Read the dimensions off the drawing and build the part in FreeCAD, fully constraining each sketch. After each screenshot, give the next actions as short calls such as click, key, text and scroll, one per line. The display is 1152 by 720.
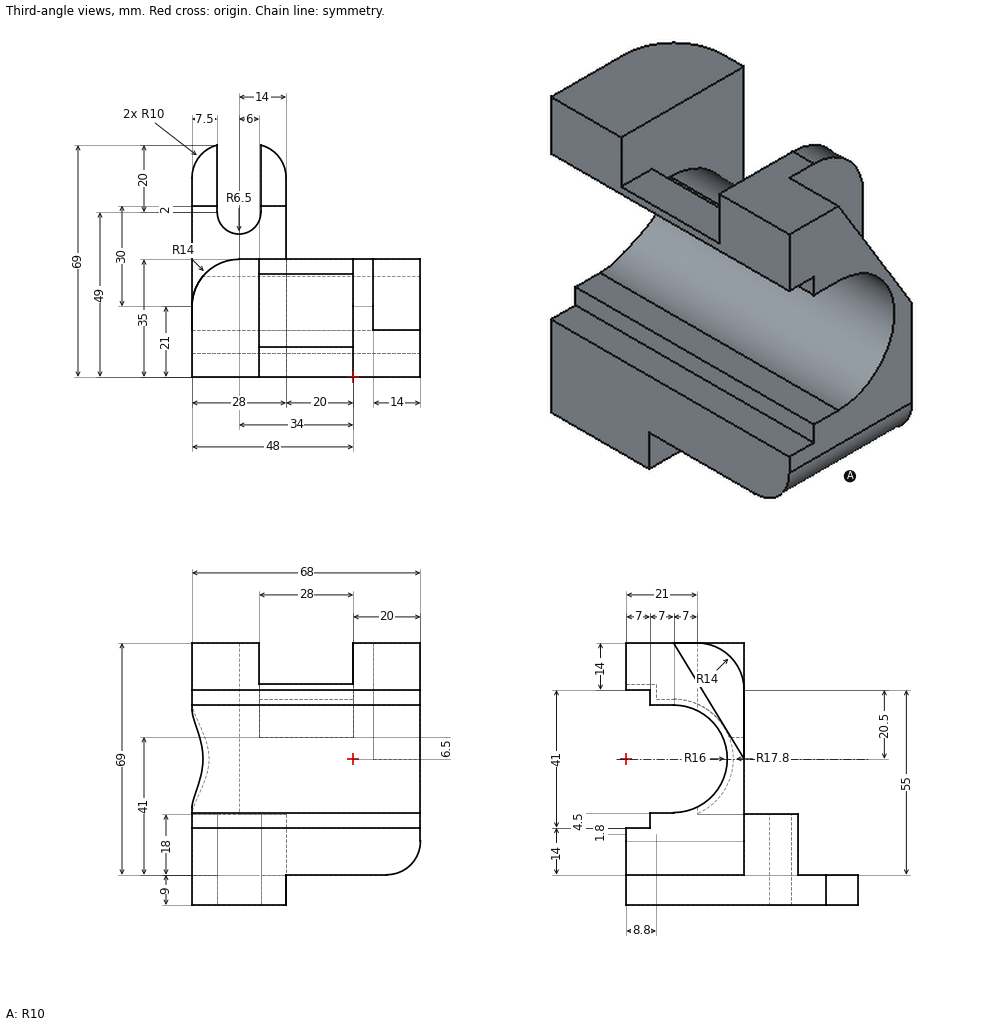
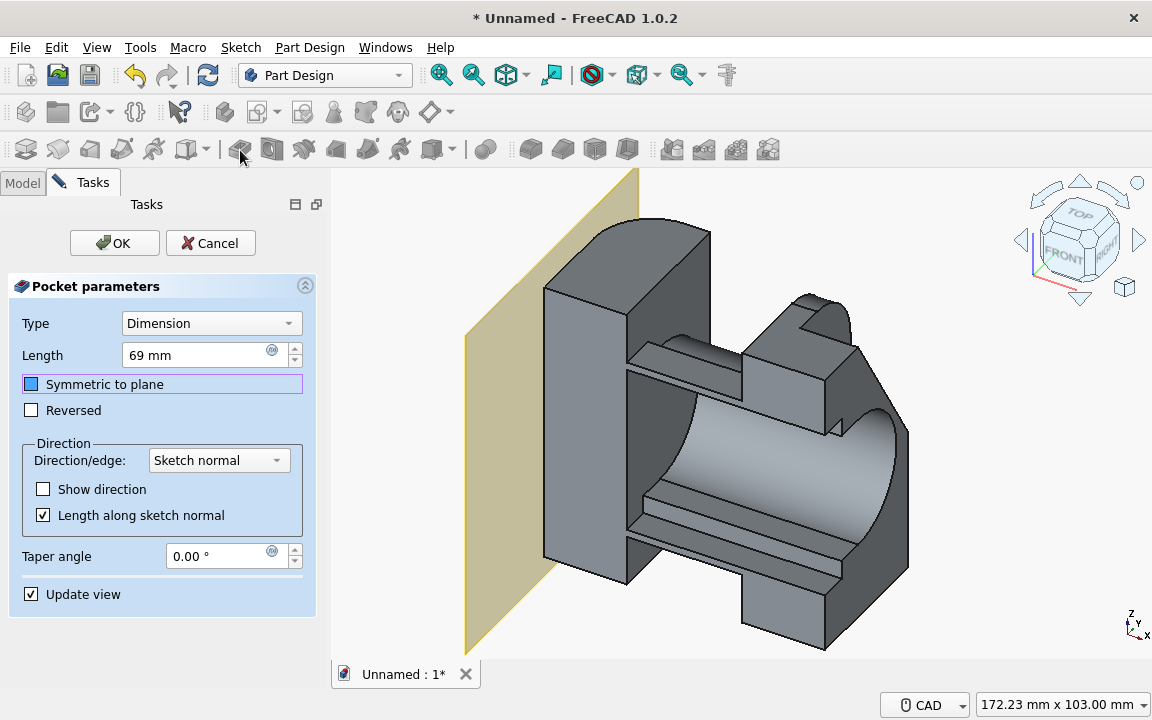
click(30, 410)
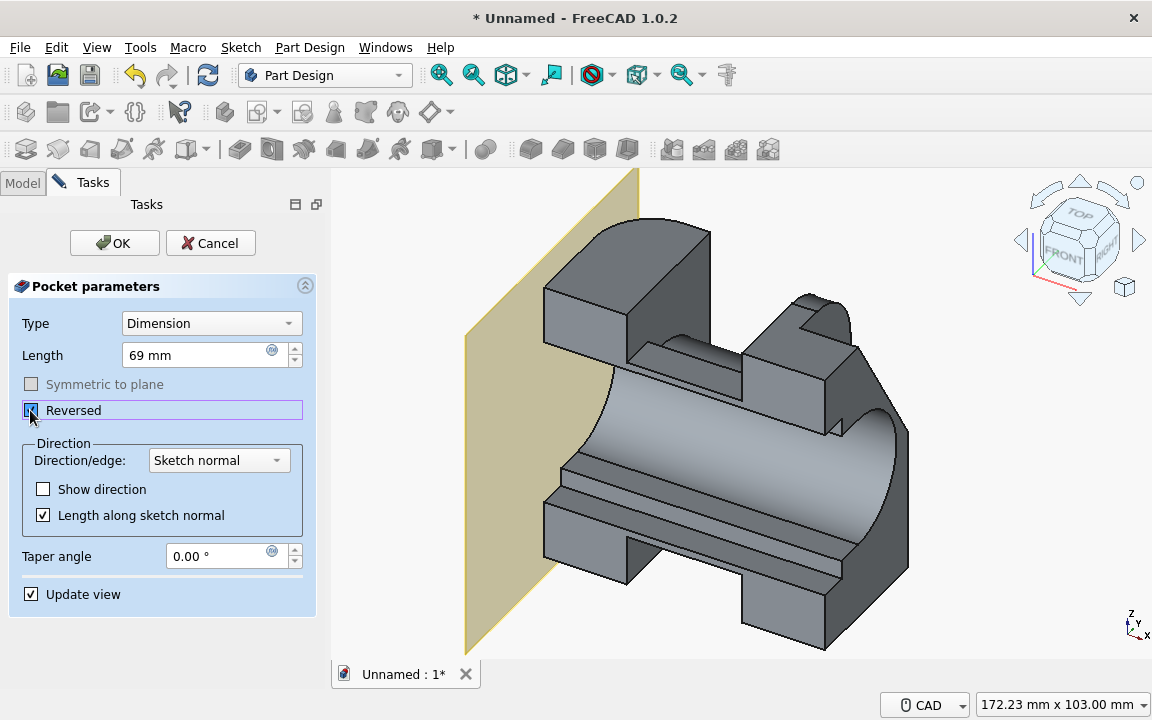
click(115, 243)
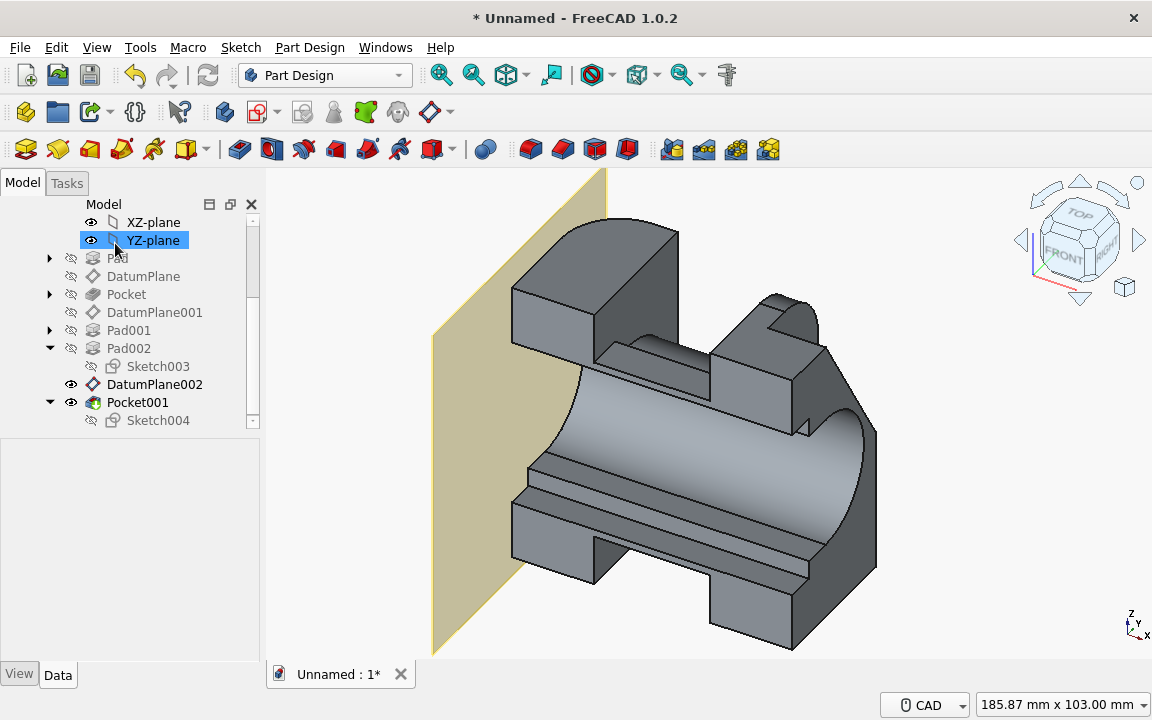
click(116, 384)
key(space)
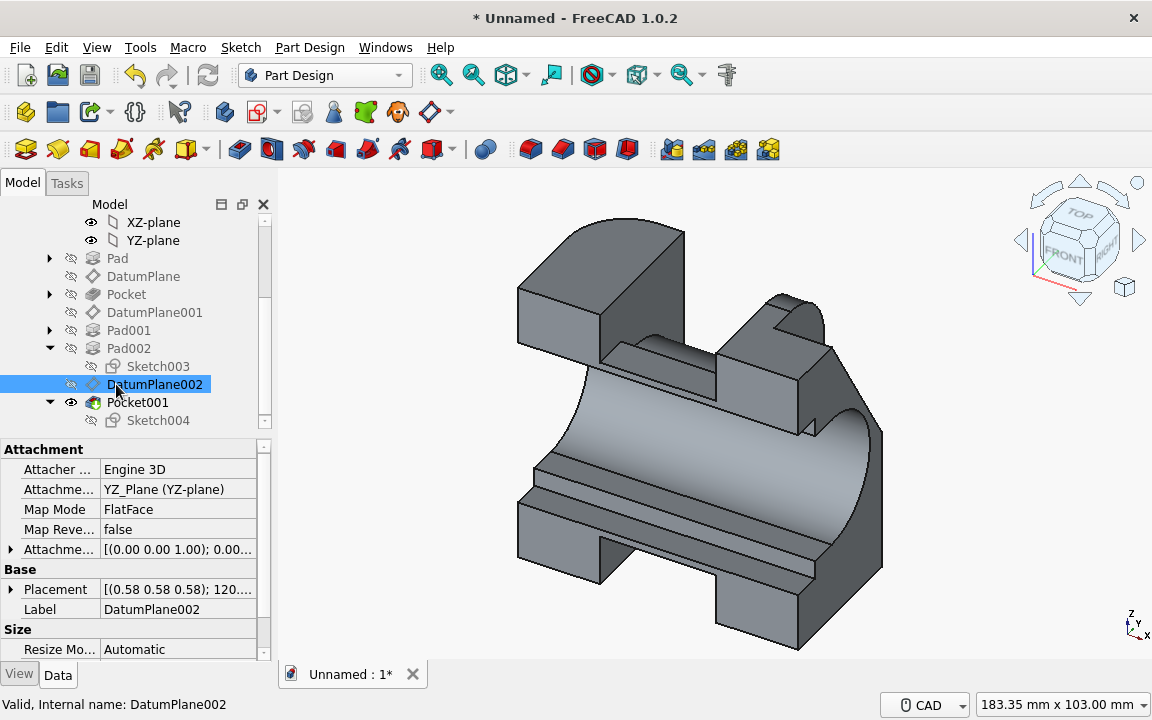
click(601, 259)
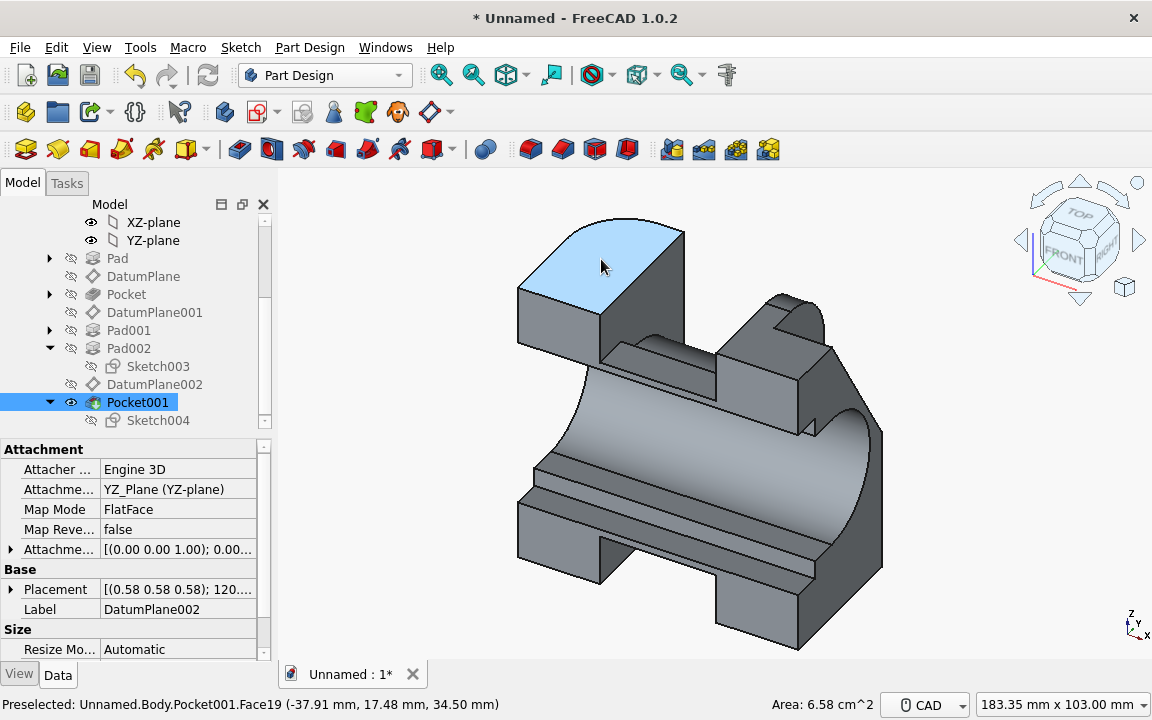
click(258, 112)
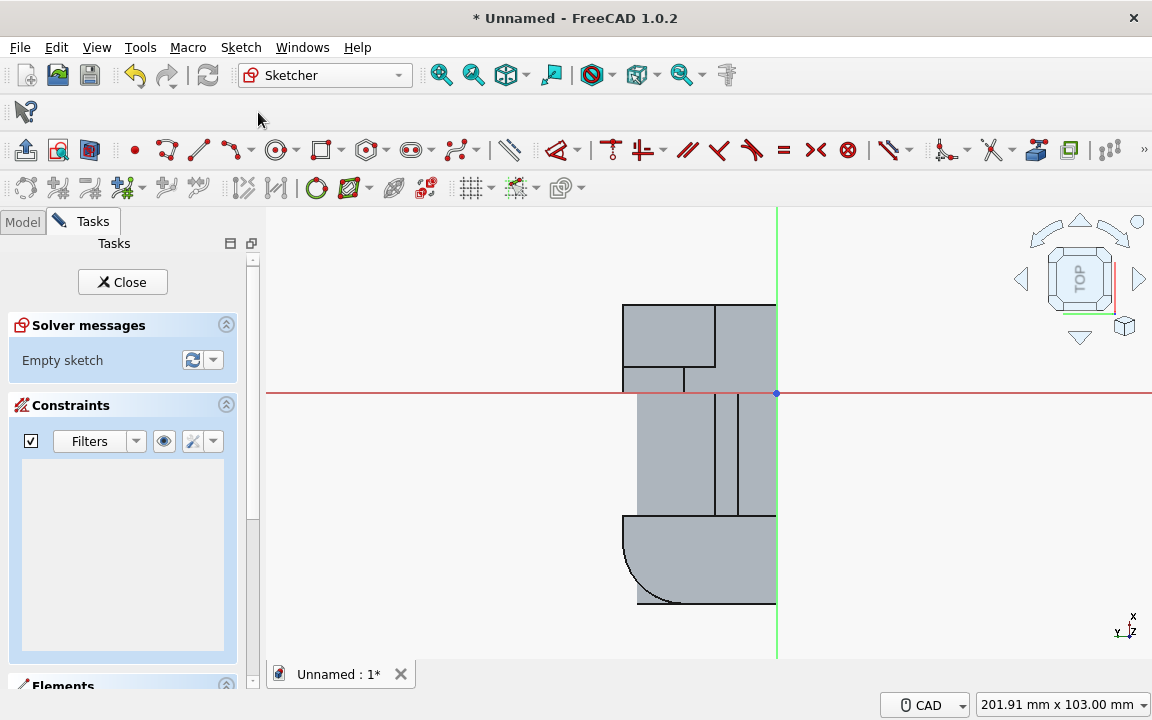
scroll(657, 608, up, 8)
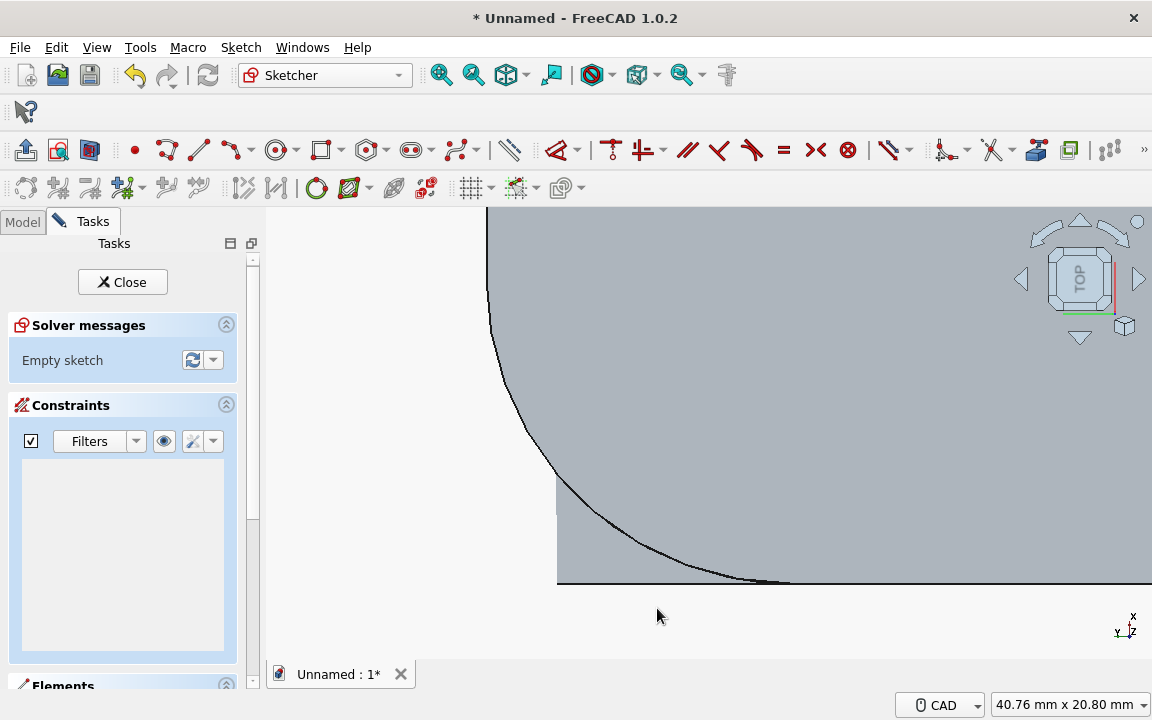
key(g)
key(m)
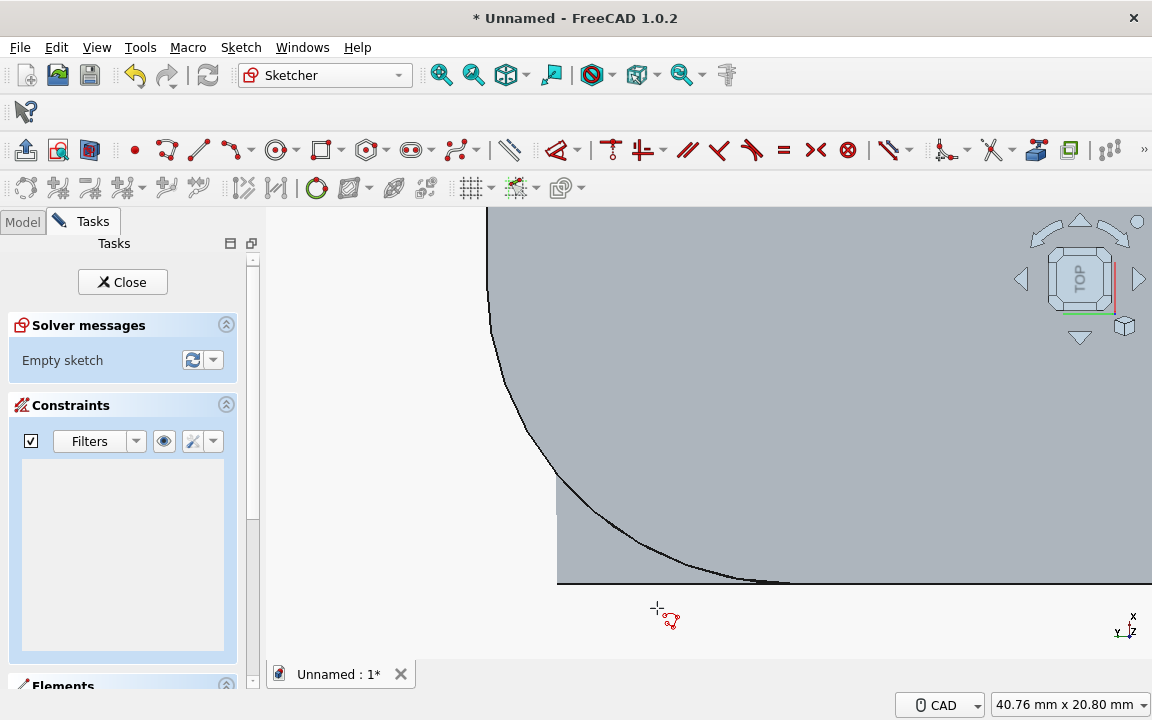
click(487, 279)
click(487, 584)
click(791, 584)
right_click(791, 584)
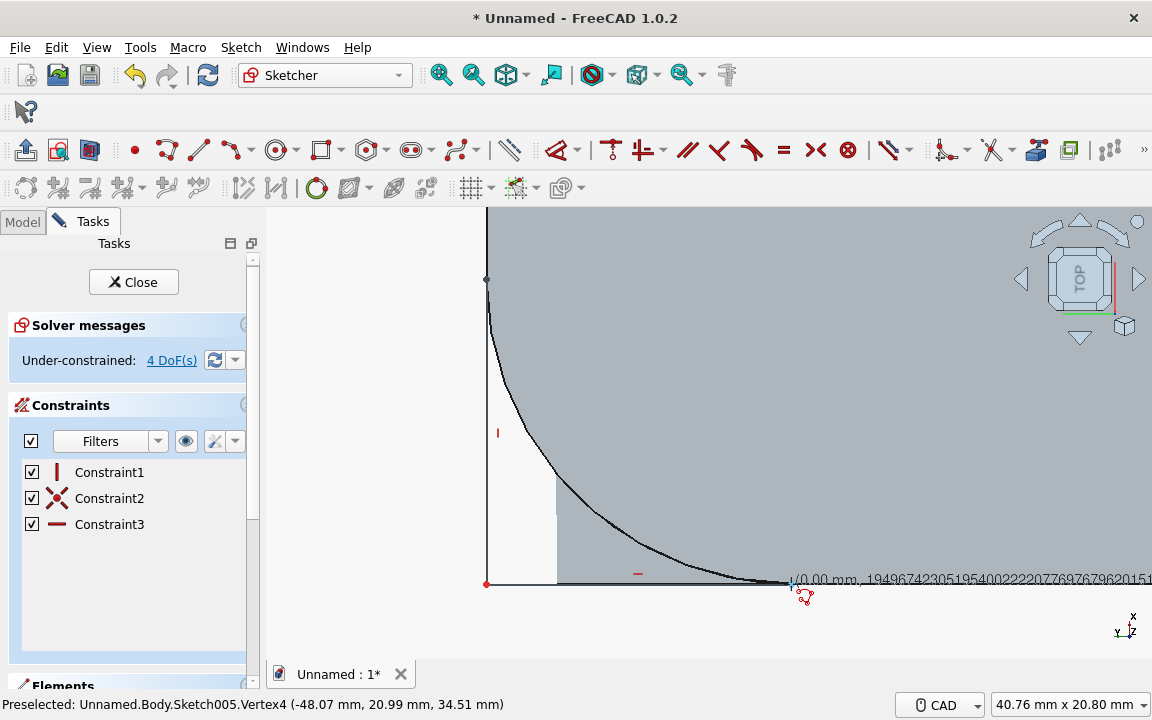
click(232, 150)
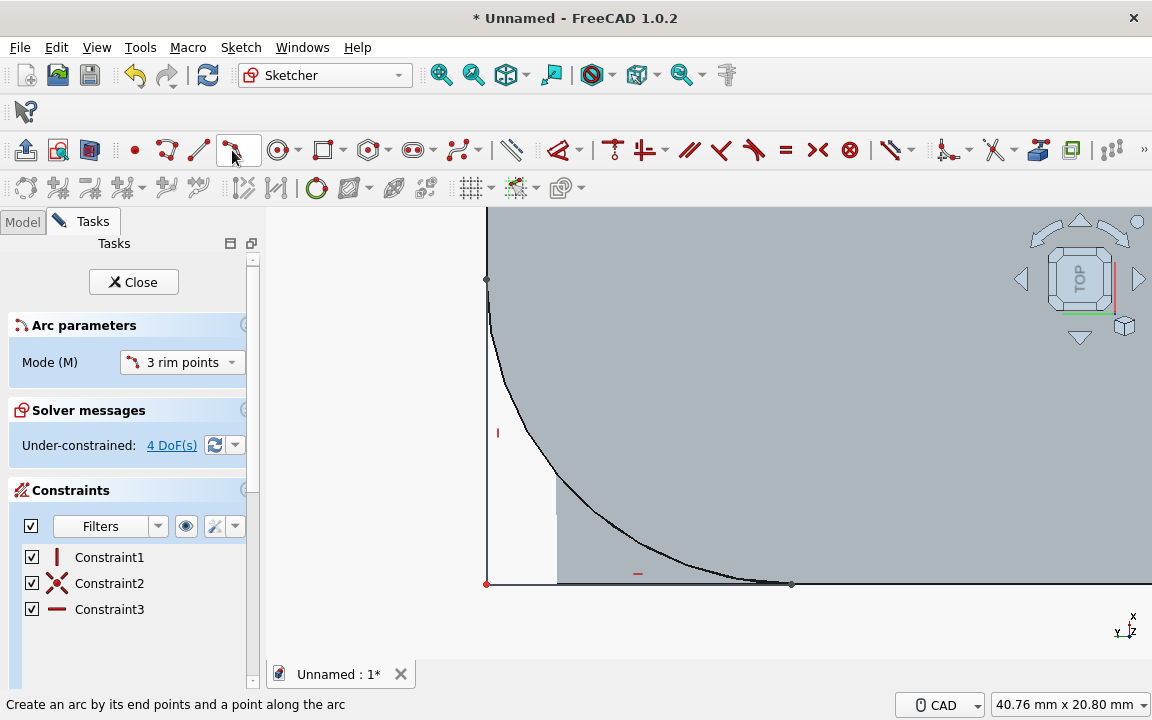
click(791, 585)
click(487, 280)
click(576, 494)
key(Escape)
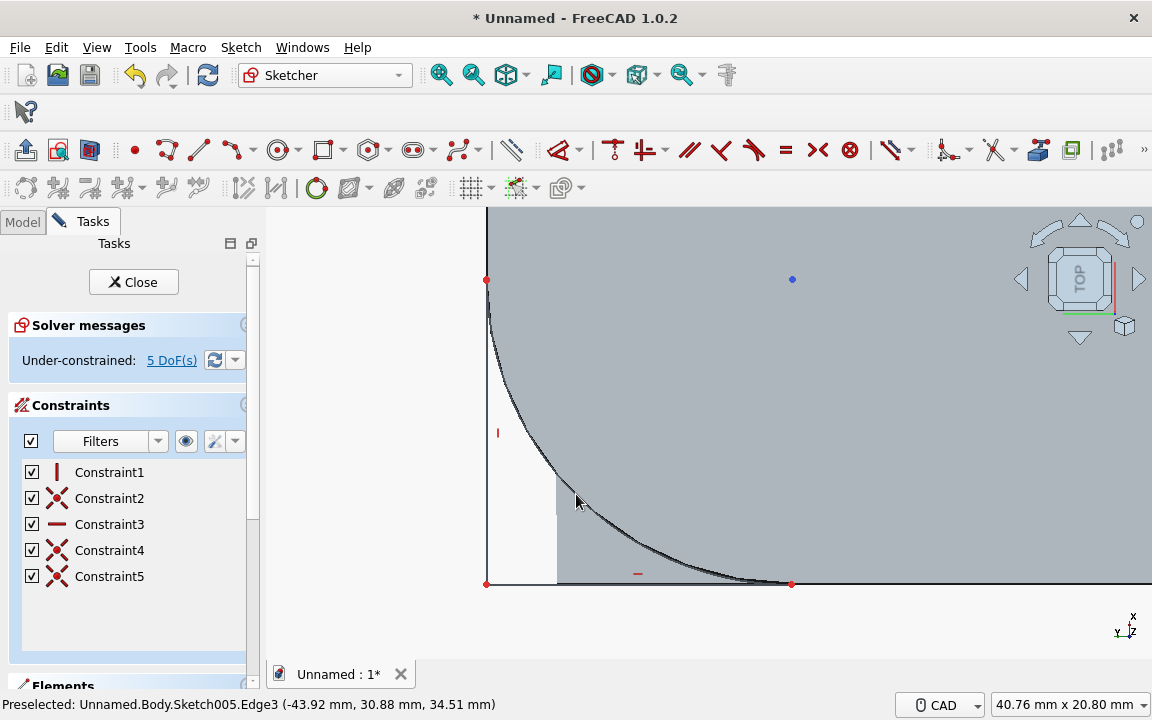
click(487, 372)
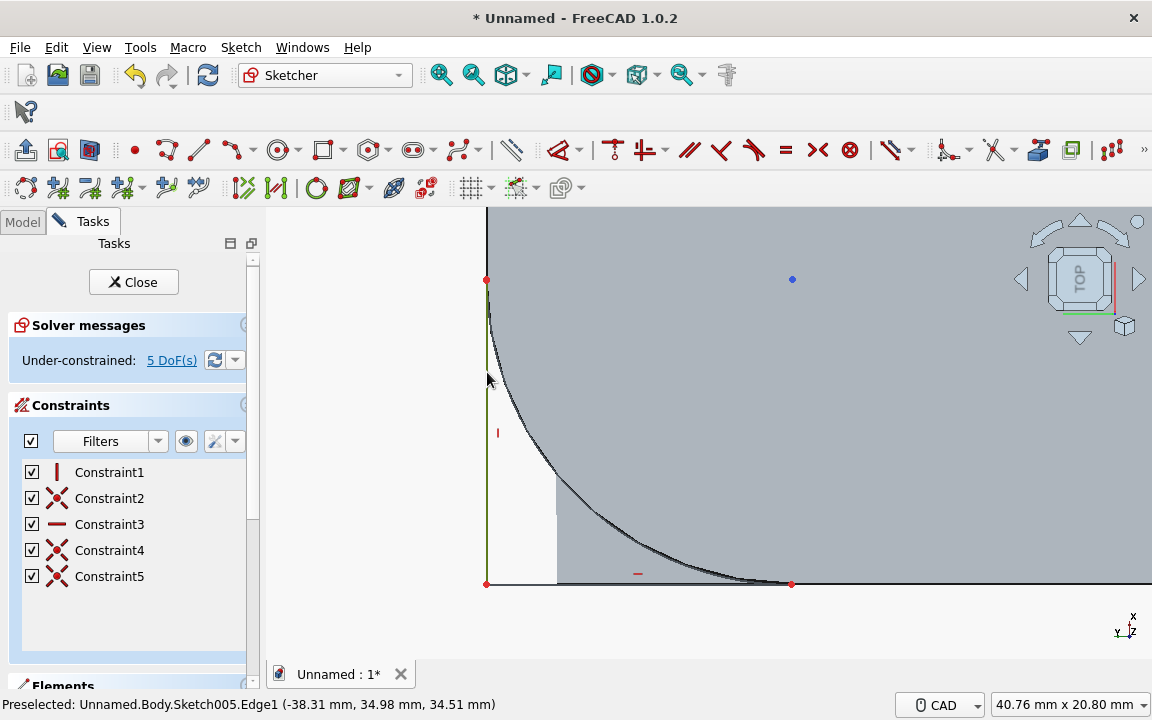
click(520, 418)